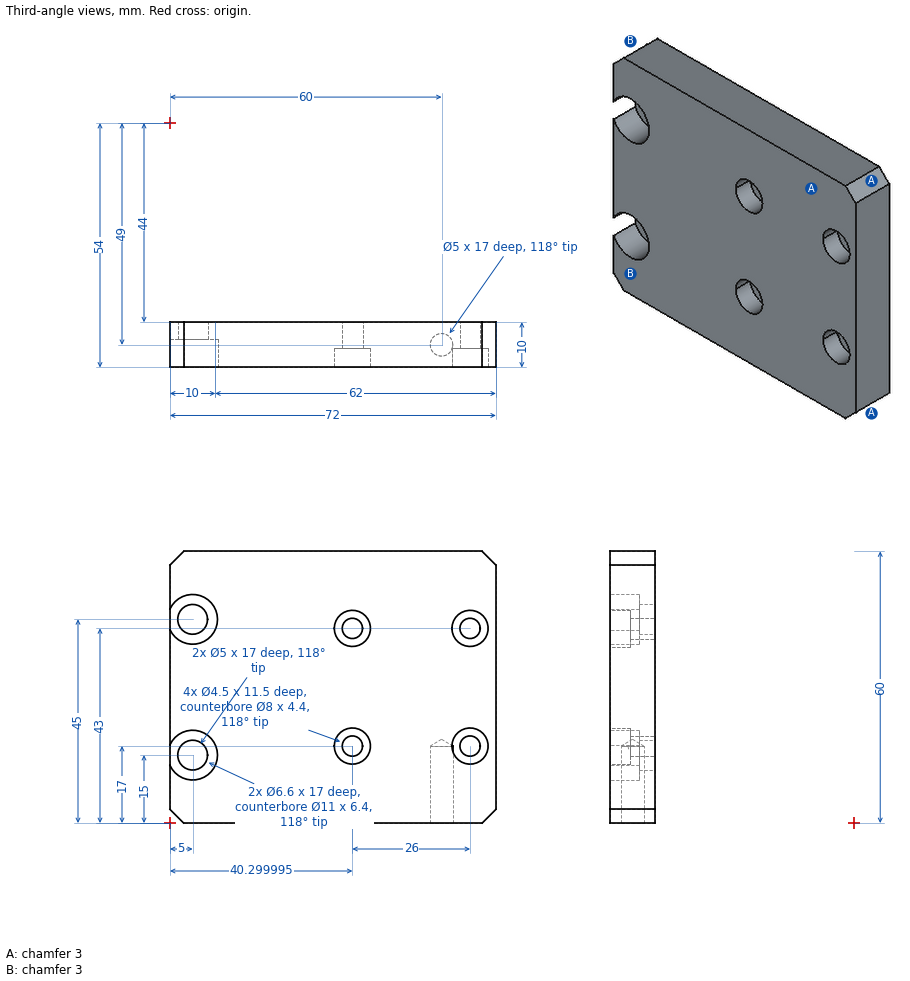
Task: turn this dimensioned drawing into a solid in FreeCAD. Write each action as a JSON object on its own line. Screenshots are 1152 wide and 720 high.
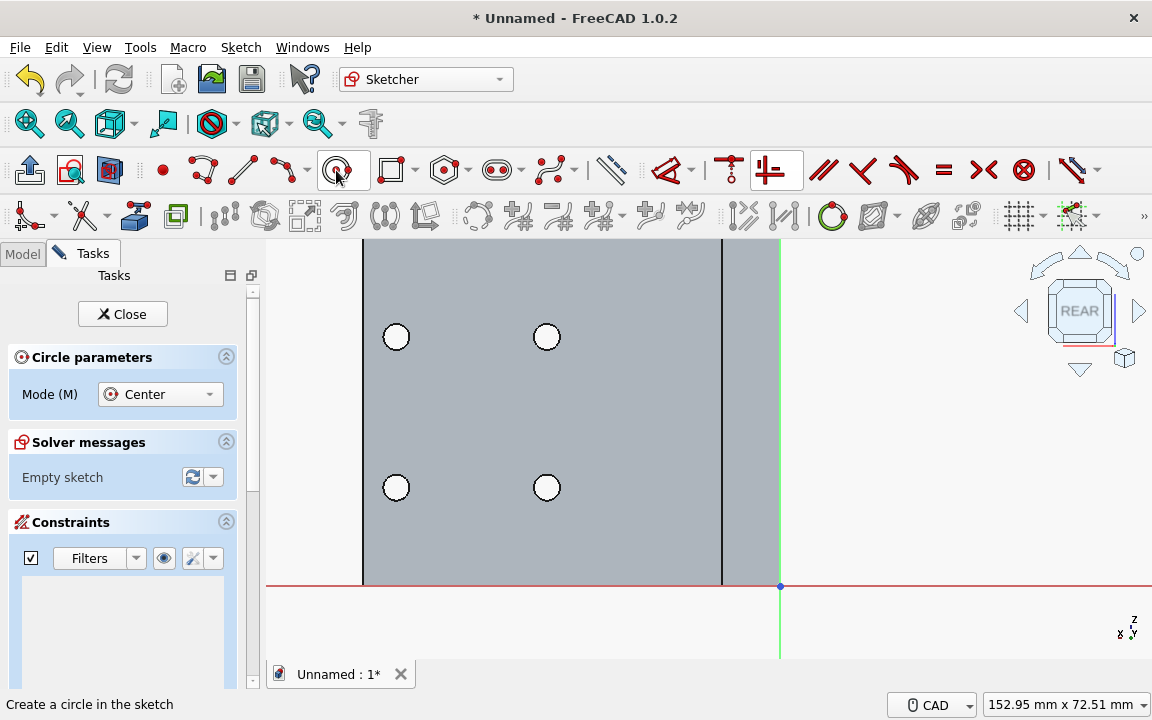
{"action": "scroll", "coordinate": [751, 499], "scroll_direction": "up", "scroll_amount": 3}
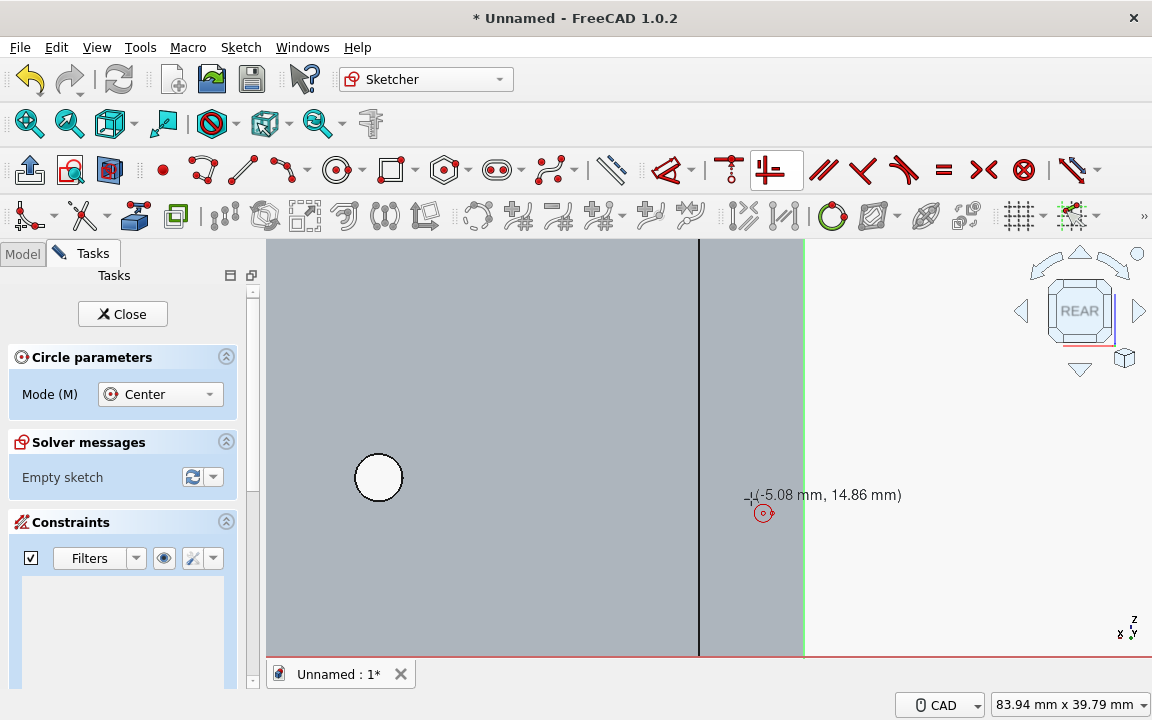
{"action": "left_click", "coordinate": [751, 499]}
{"action": "left_click", "coordinate": [770, 480]}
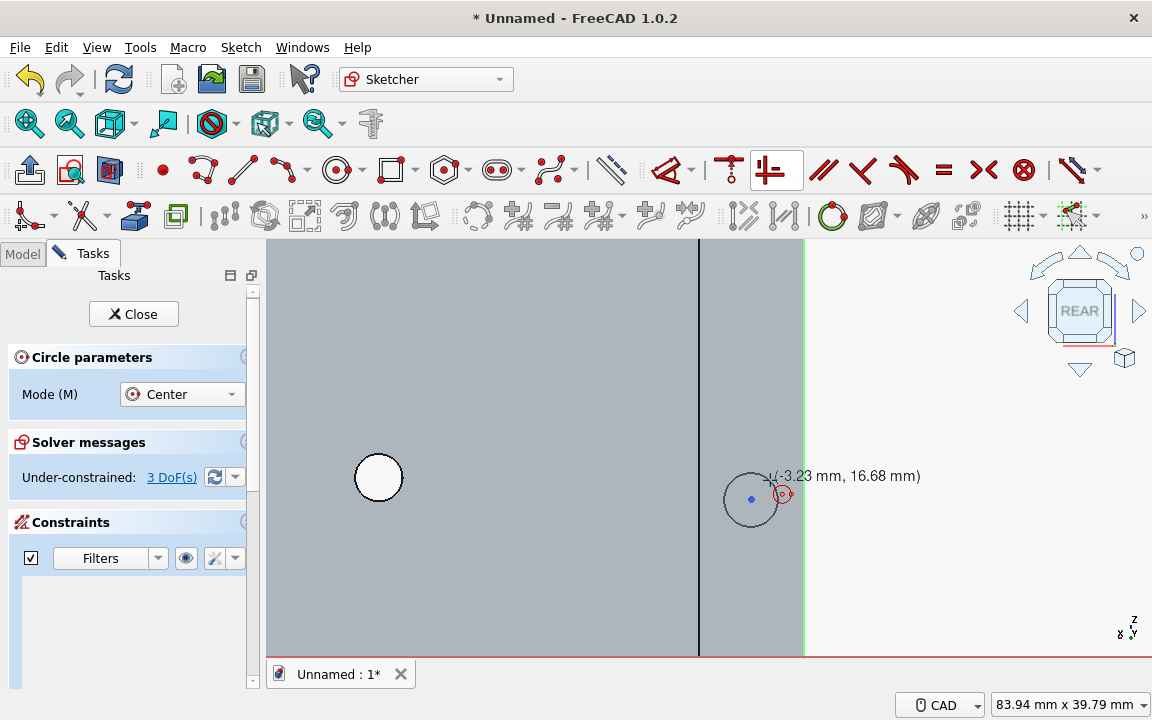
{"action": "scroll", "coordinate": [490, 501], "scroll_direction": "down", "scroll_amount": 3}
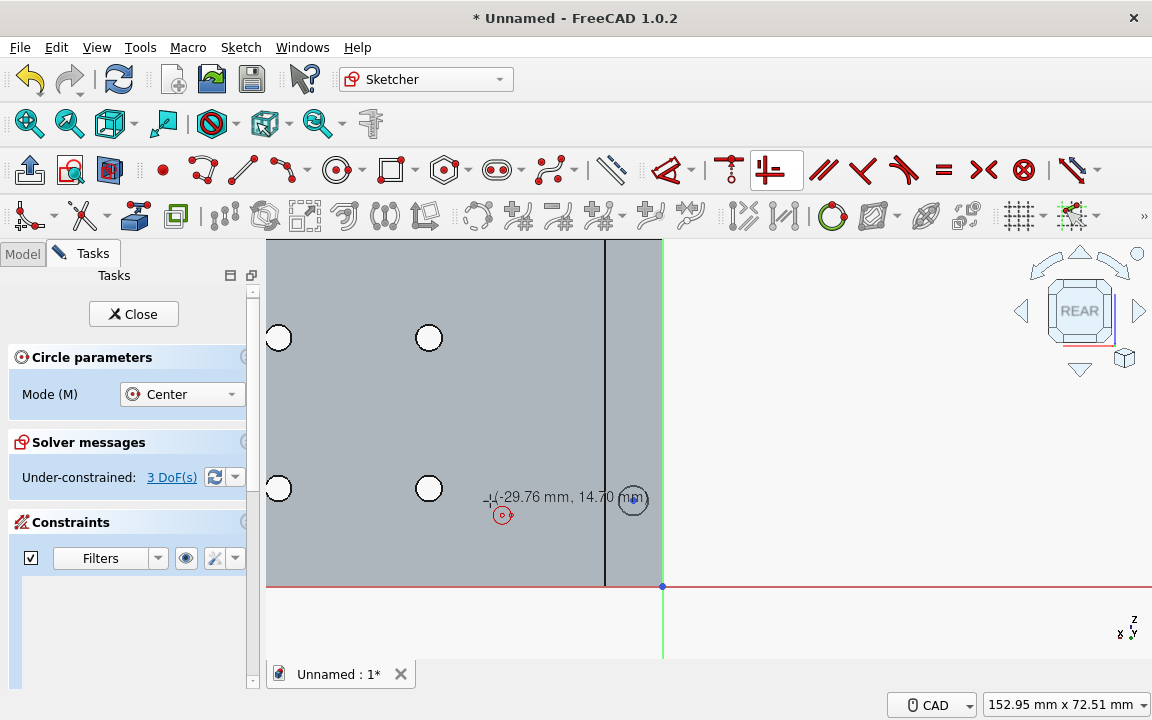
{"action": "scroll", "coordinate": [634, 326], "scroll_direction": "up", "scroll_amount": 3}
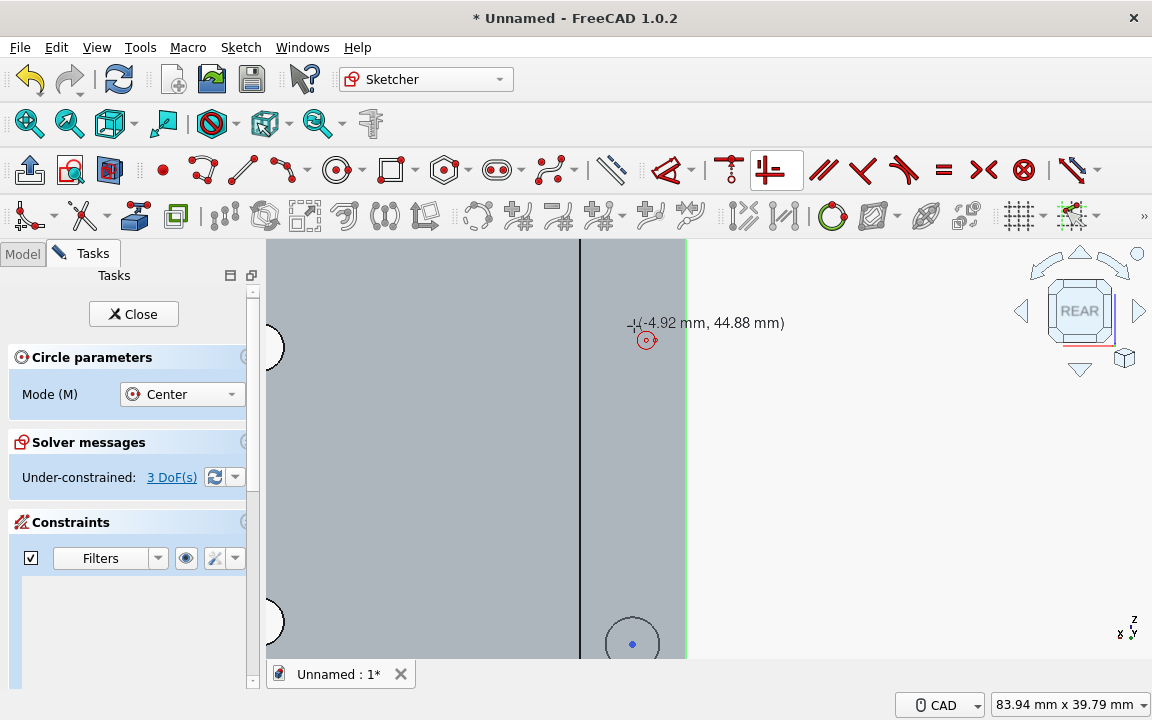
{"action": "left_click", "coordinate": [633, 326]}
{"action": "left_click", "coordinate": [651, 308]}
{"action": "key", "text": "Escape"}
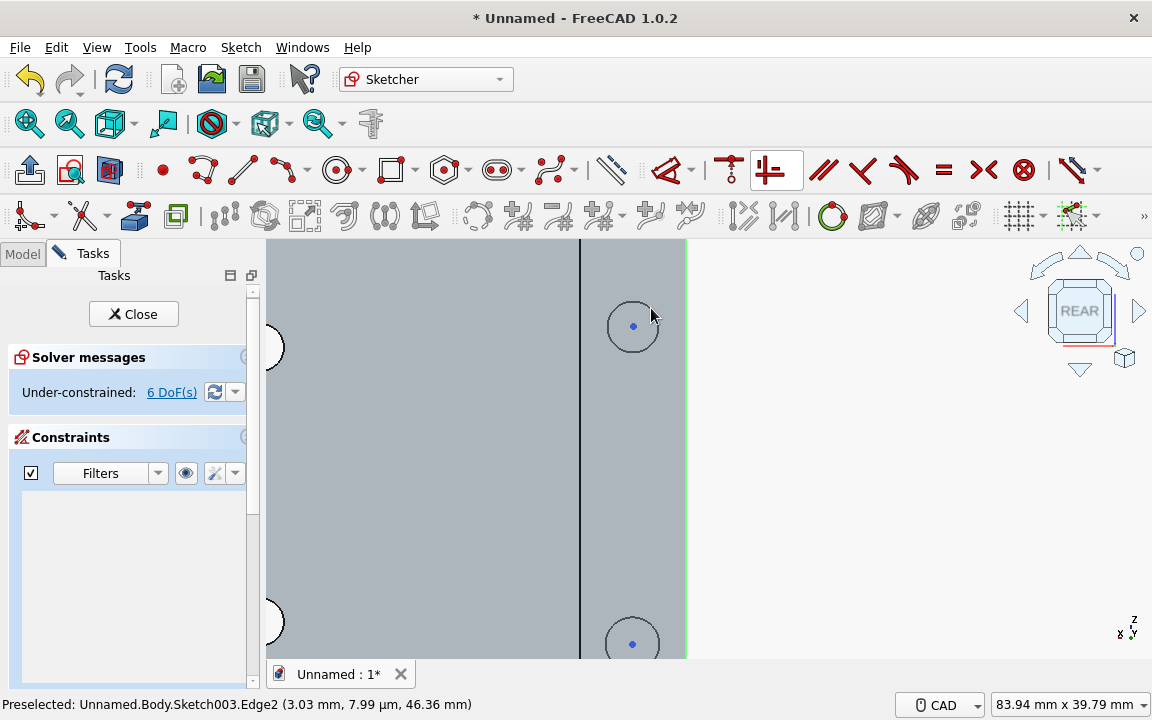
{"action": "left_click", "coordinate": [651, 625]}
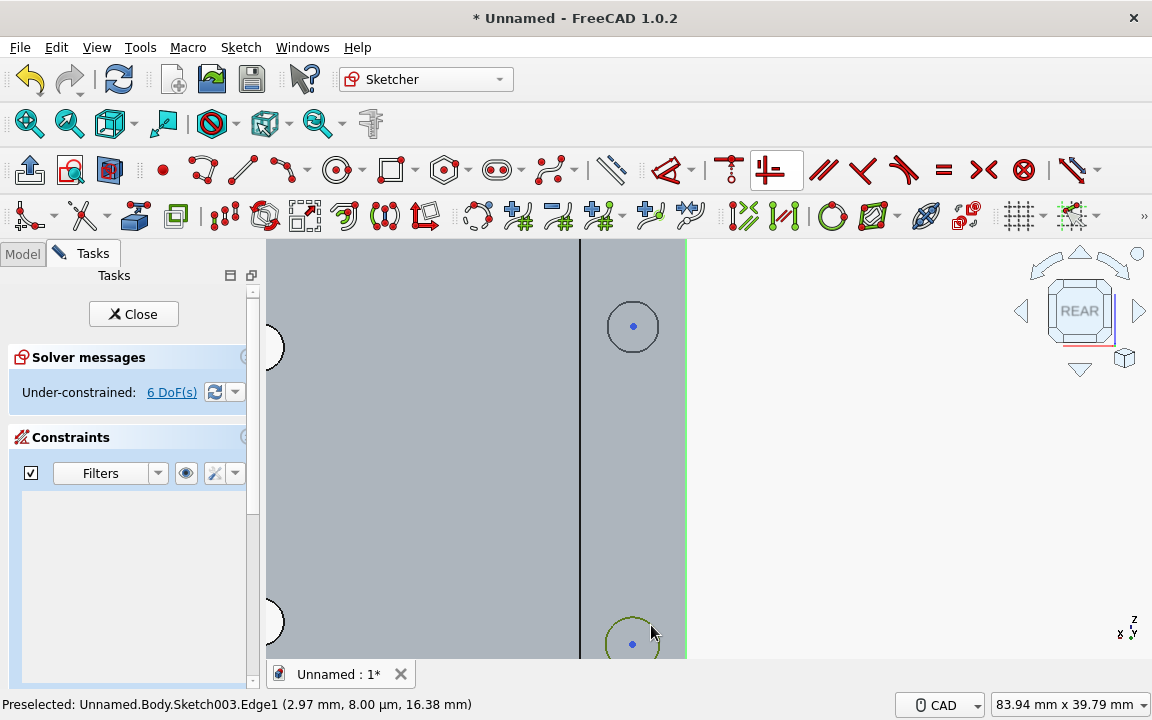
{"action": "left_click", "coordinate": [651, 309]}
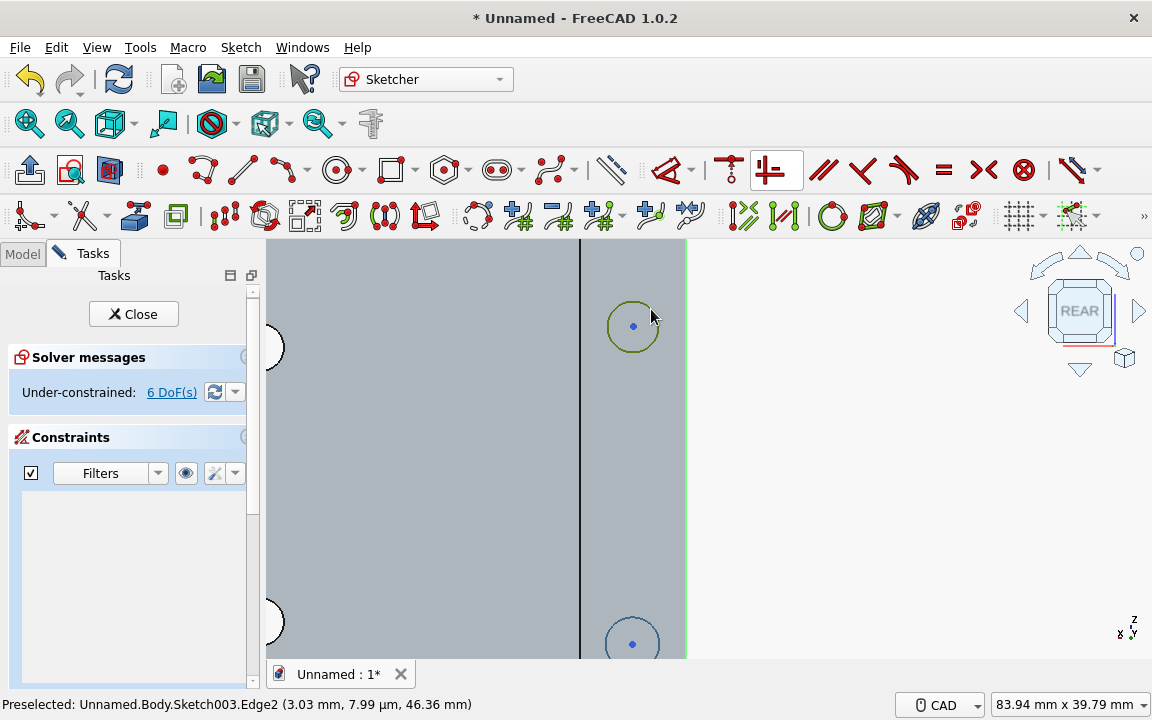
{"action": "left_click", "coordinate": [944, 170]}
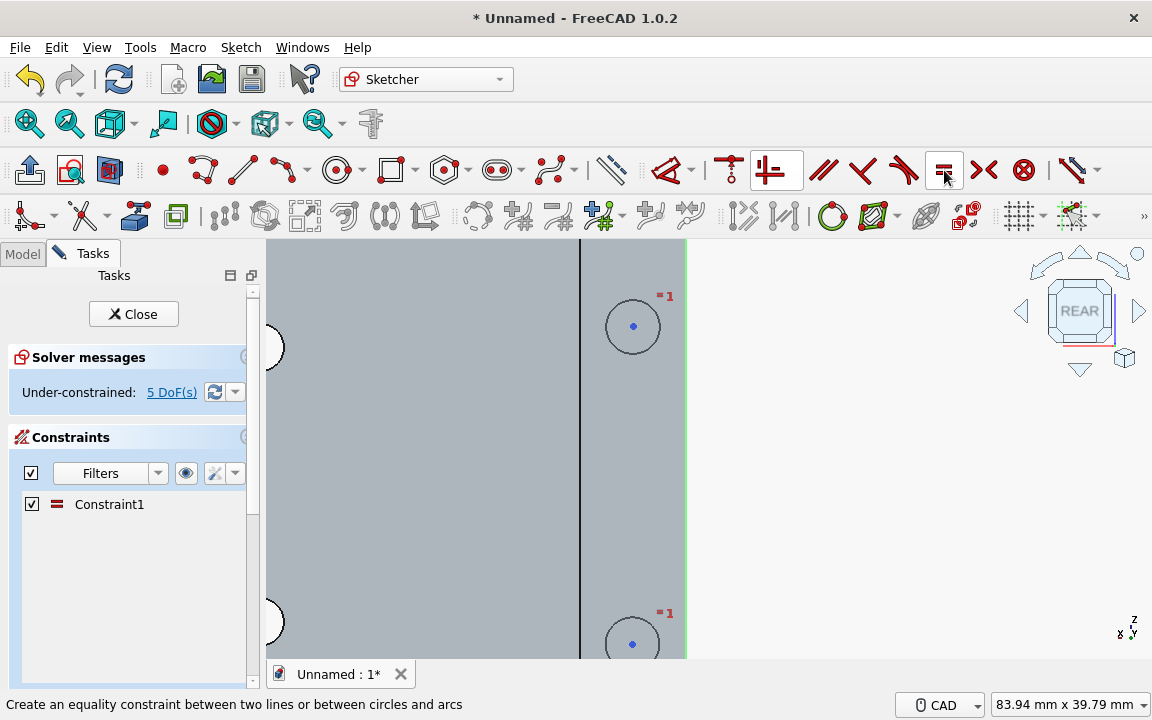
{"action": "scroll", "coordinate": [634, 325], "scroll_direction": "down", "scroll_amount": 3}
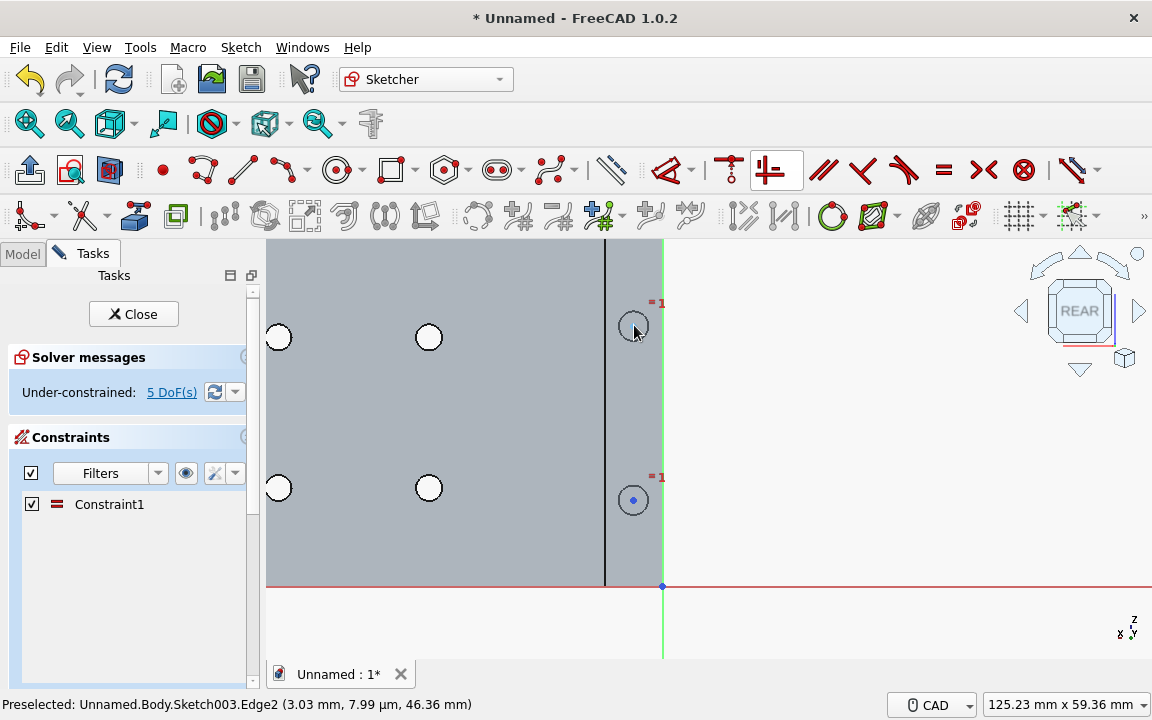
{"action": "left_click", "coordinate": [633, 500]}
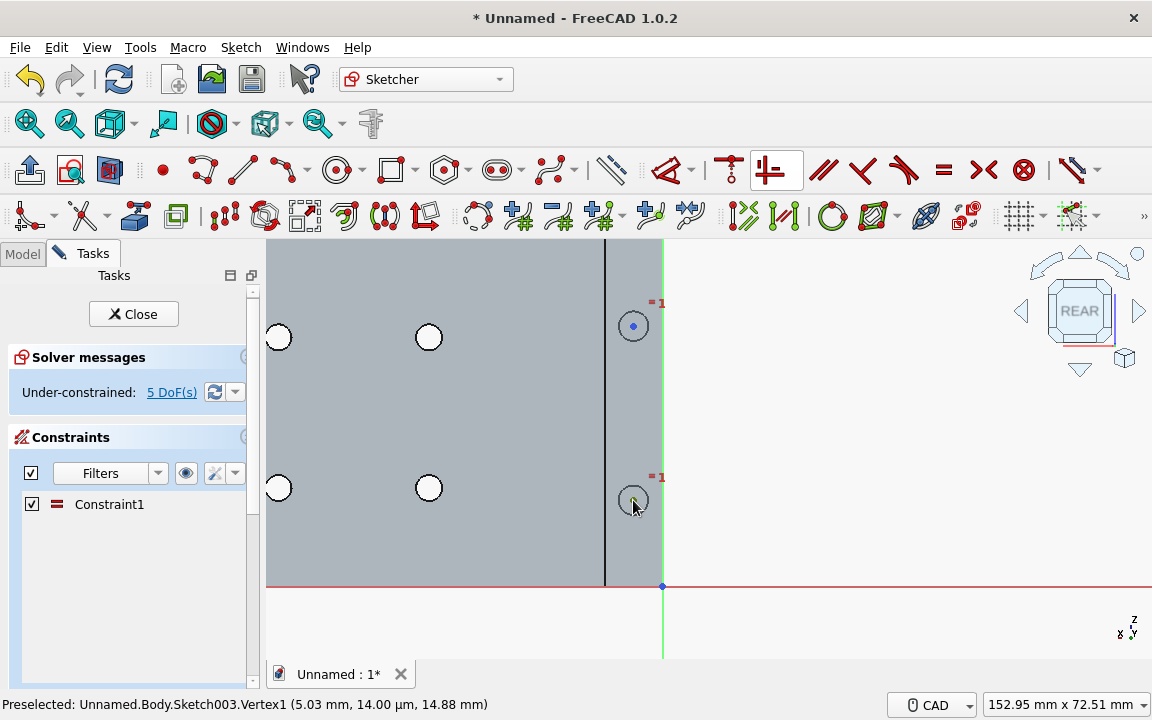
{"action": "left_click", "coordinate": [634, 326]}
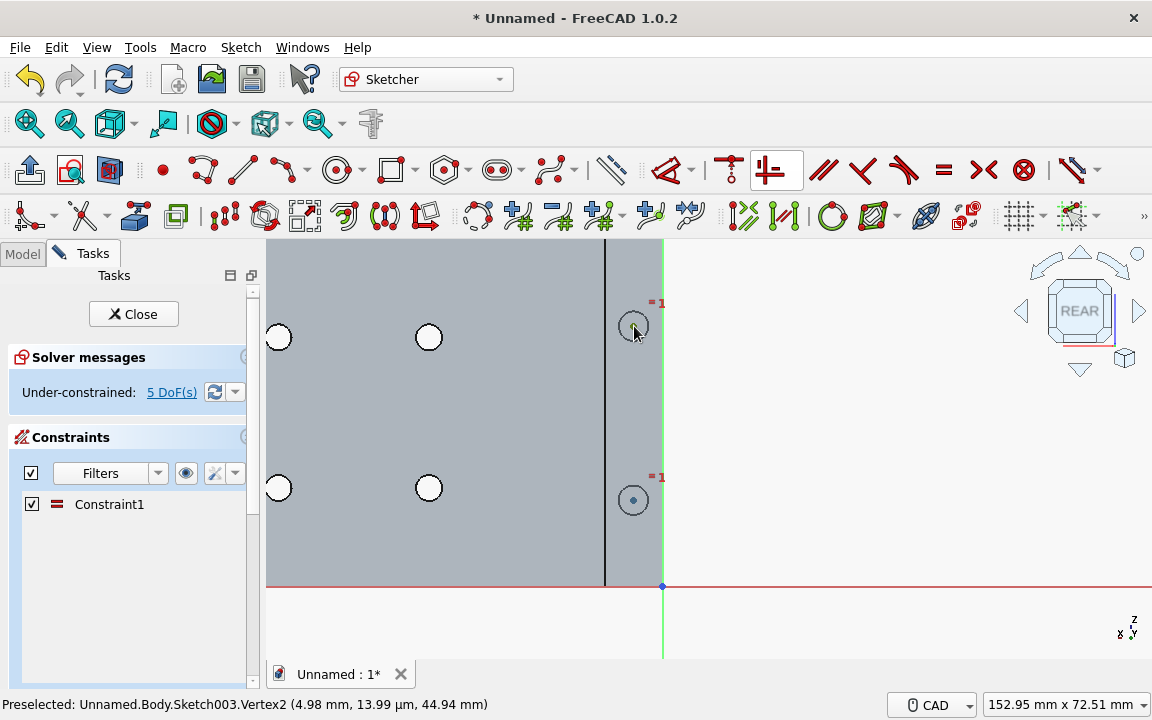
{"action": "key", "text": "v"}